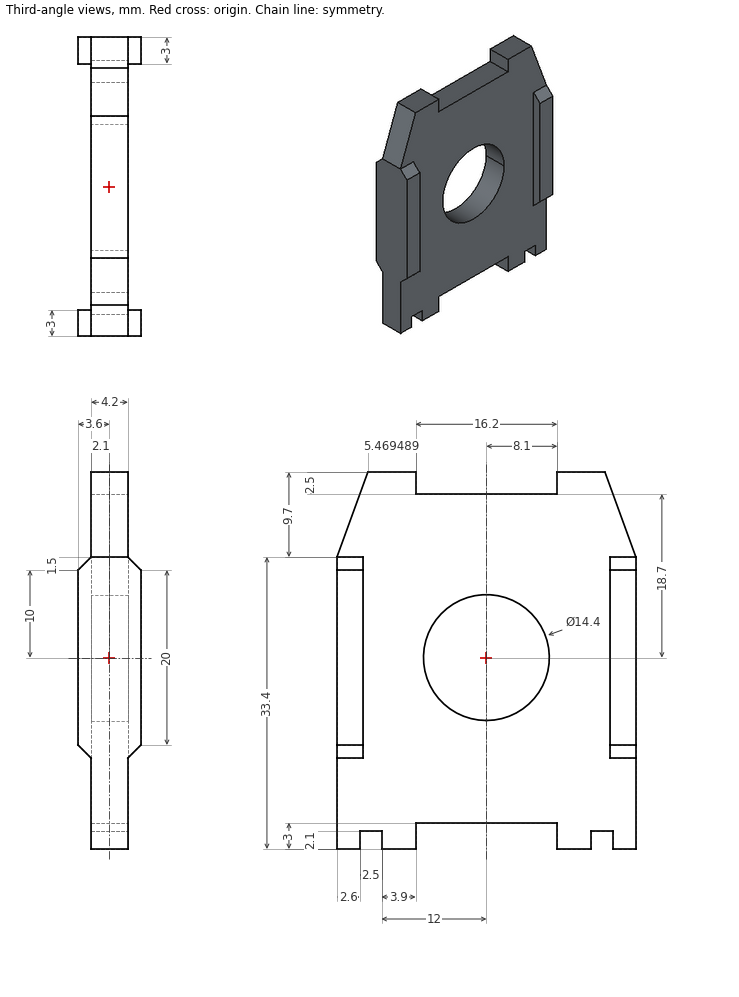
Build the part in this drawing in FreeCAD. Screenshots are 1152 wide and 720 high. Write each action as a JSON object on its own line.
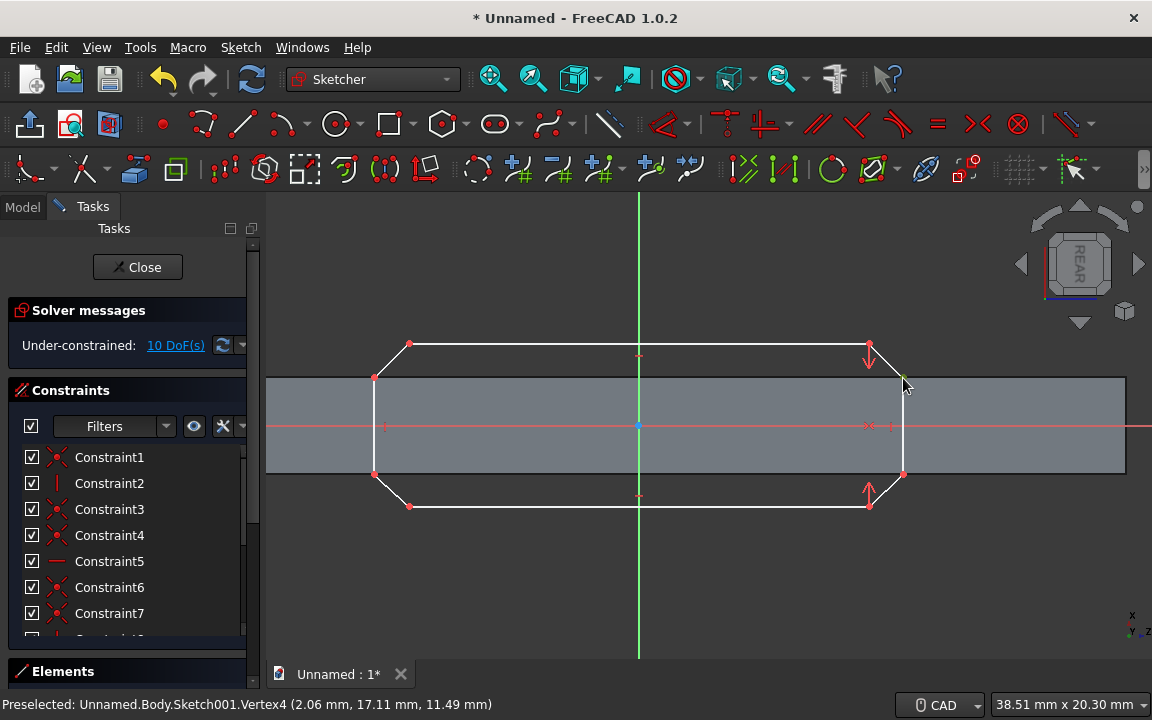
{"action": "left_click", "coordinate": [374, 378]}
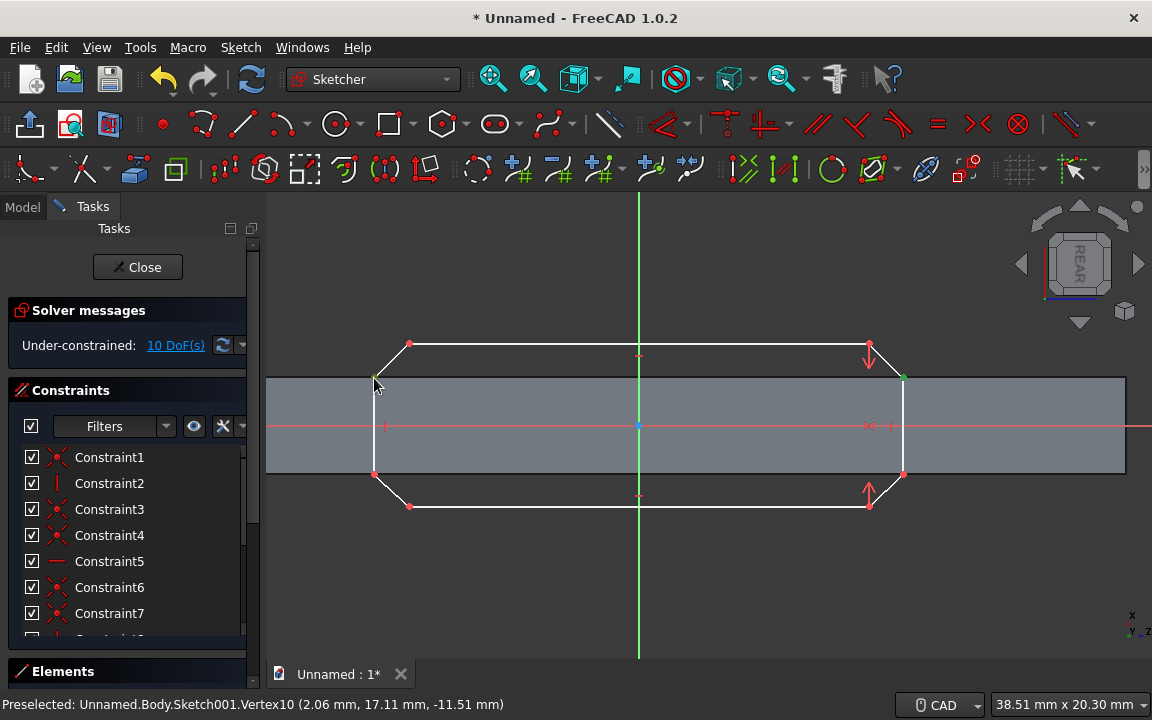
{"action": "left_click", "coordinate": [639, 602]}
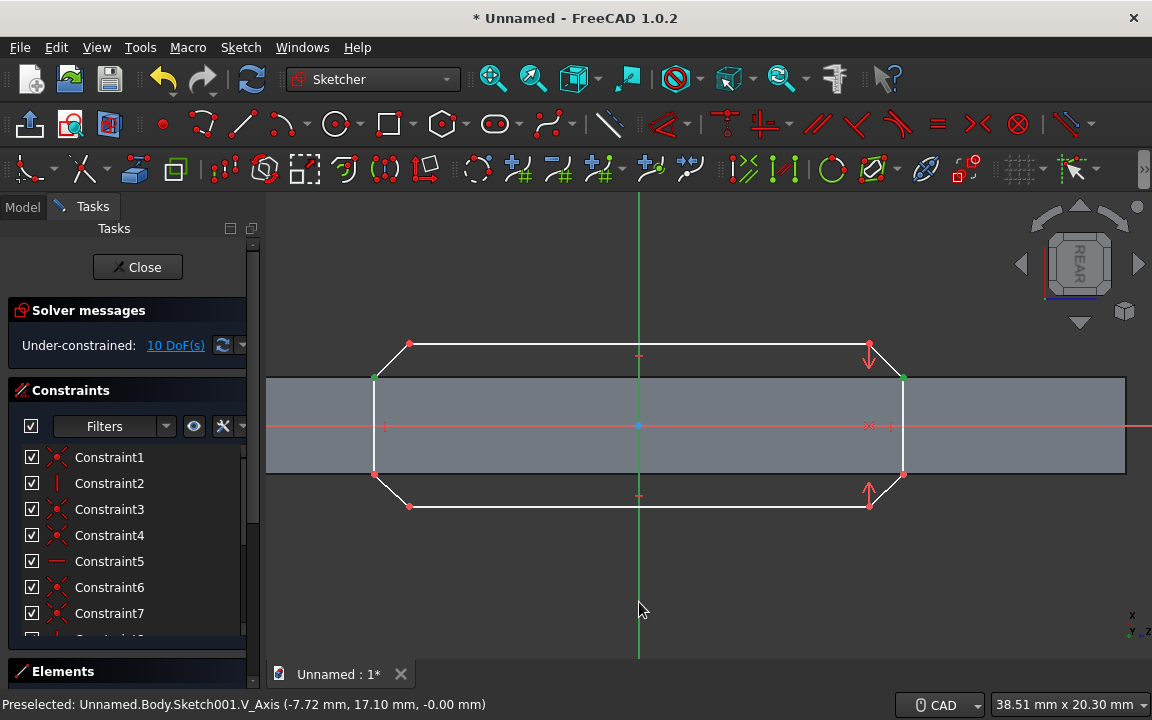
{"action": "key", "text": "s"}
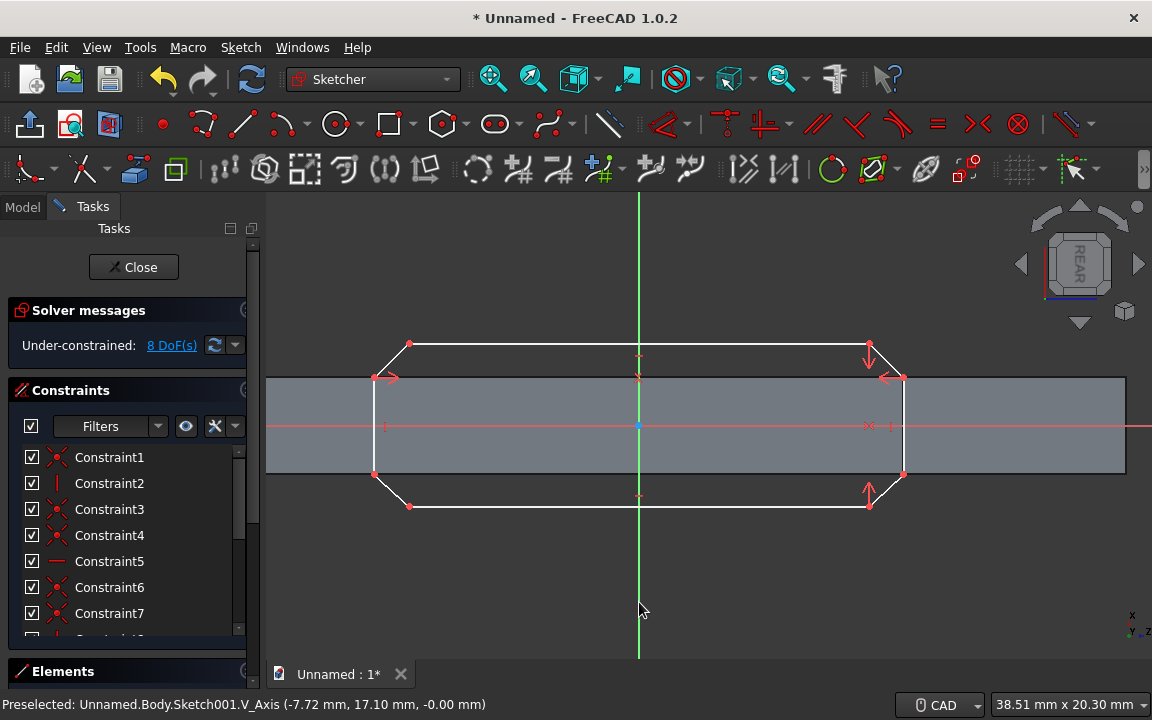
{"action": "left_click", "coordinate": [664, 124]}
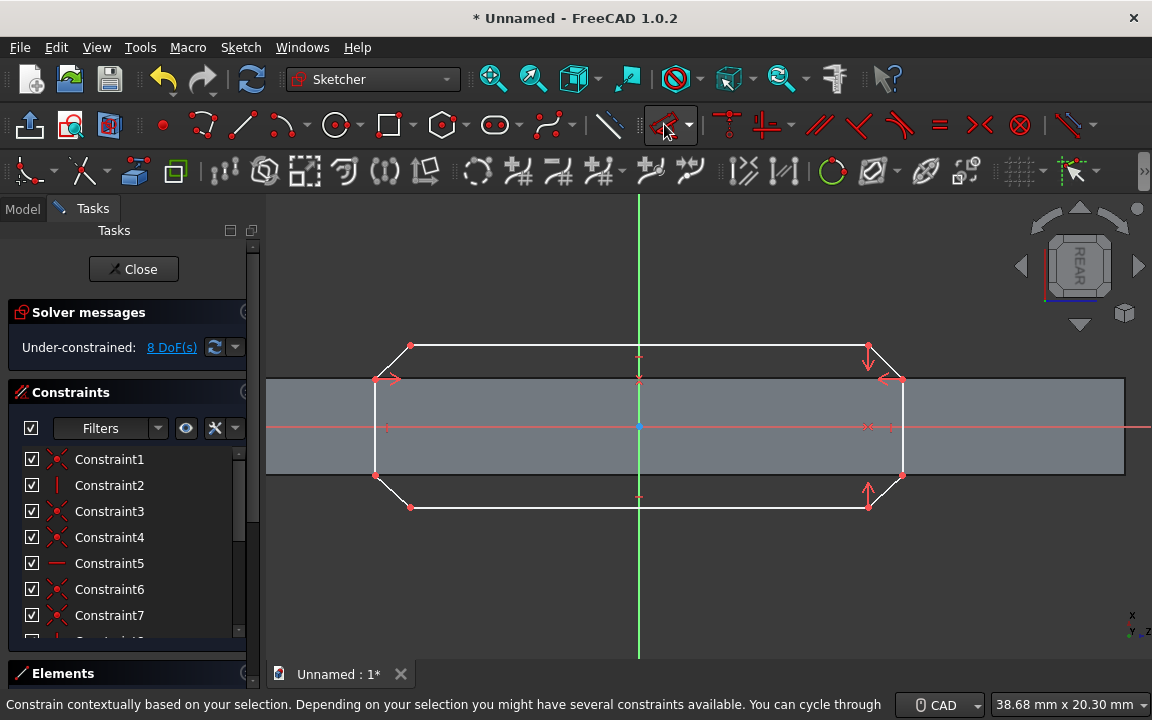
{"action": "left_click", "coordinate": [731, 345]}
{"action": "left_click", "coordinate": [534, 311]}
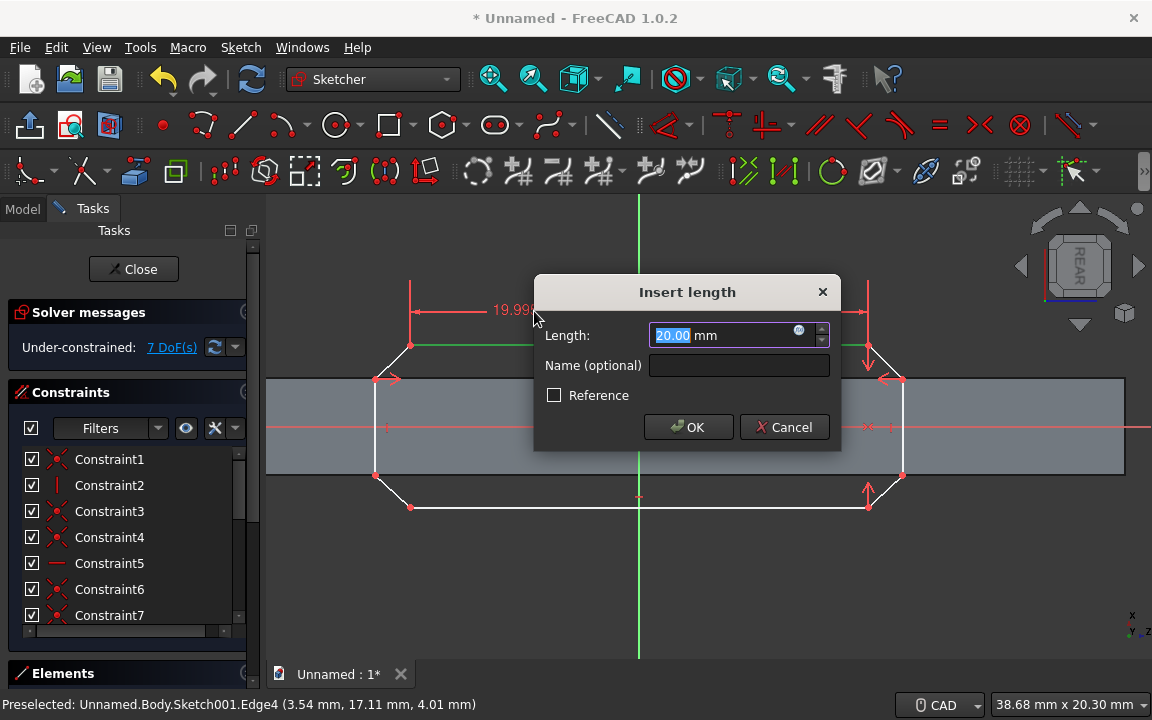
{"action": "type", "text": "20"}
{"action": "key", "text": "Return"}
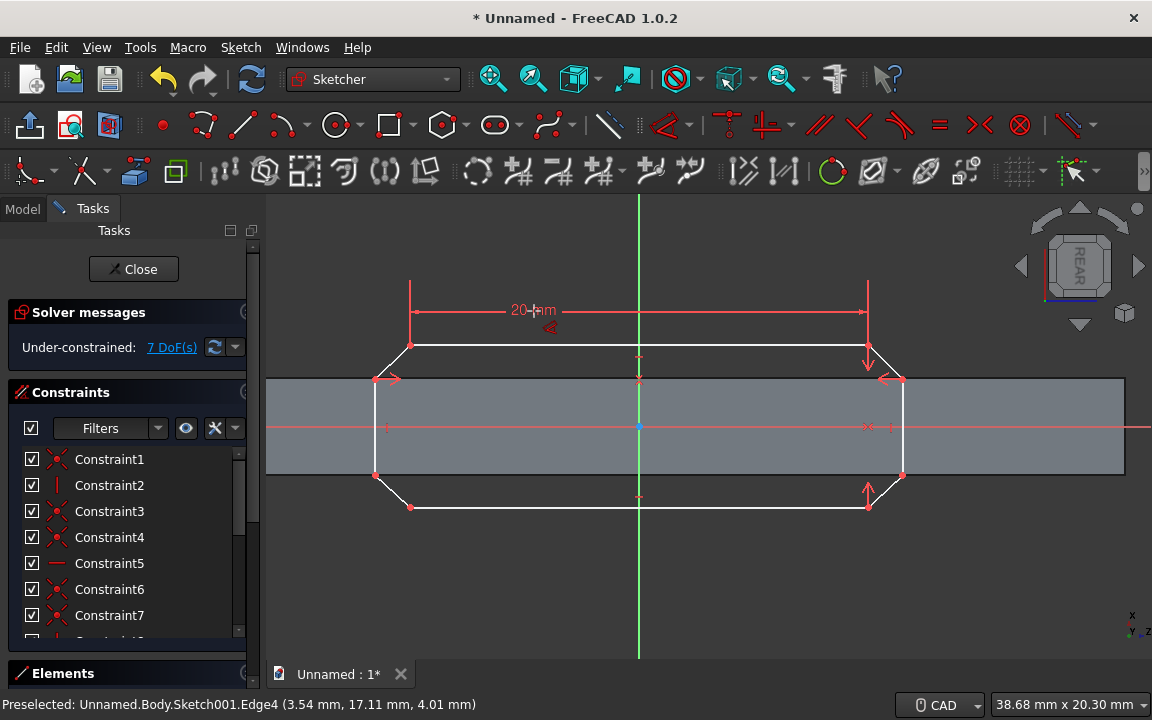
{"action": "left_click", "coordinate": [548, 508]}
{"action": "left_click", "coordinate": [534, 542]}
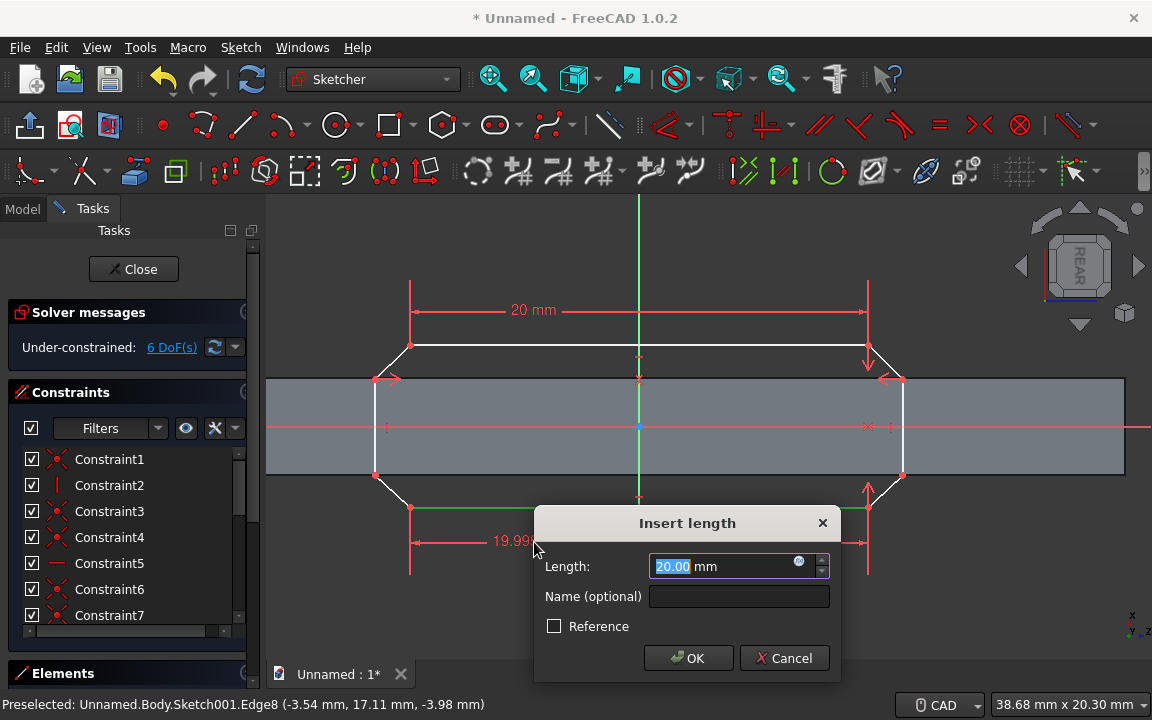
{"action": "type", "text": "20"}
{"action": "key", "text": "Return"}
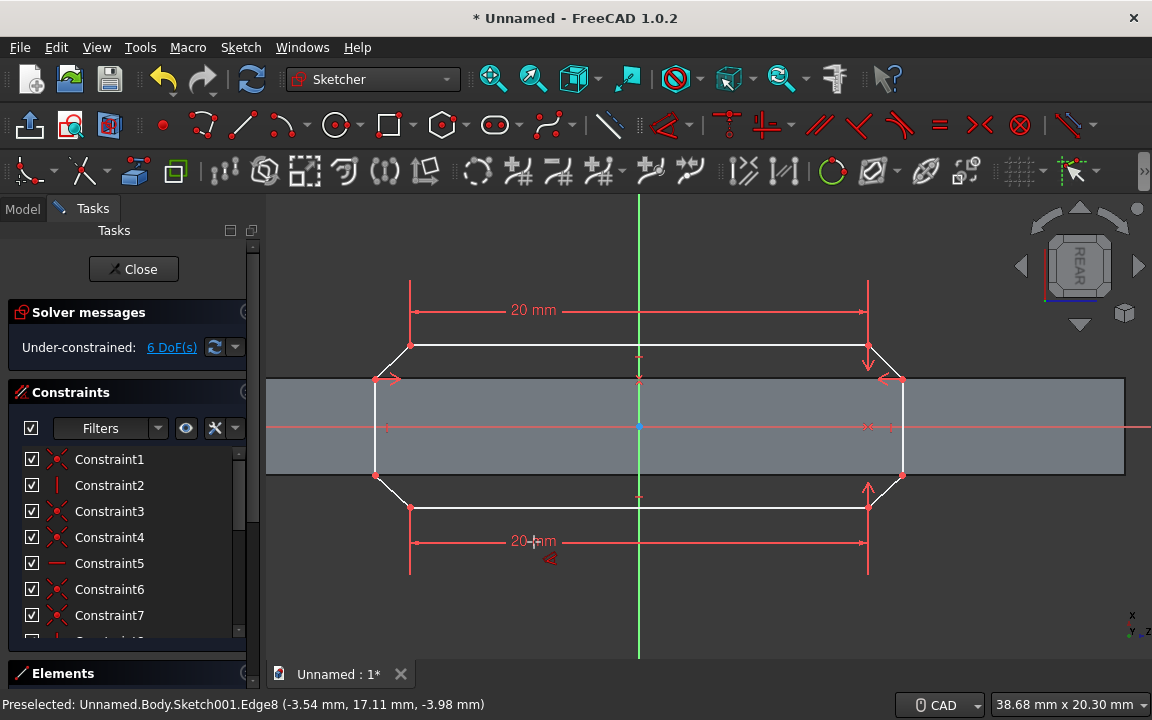
{"action": "left_click", "coordinate": [903, 447]}
{"action": "left_click", "coordinate": [937, 405]}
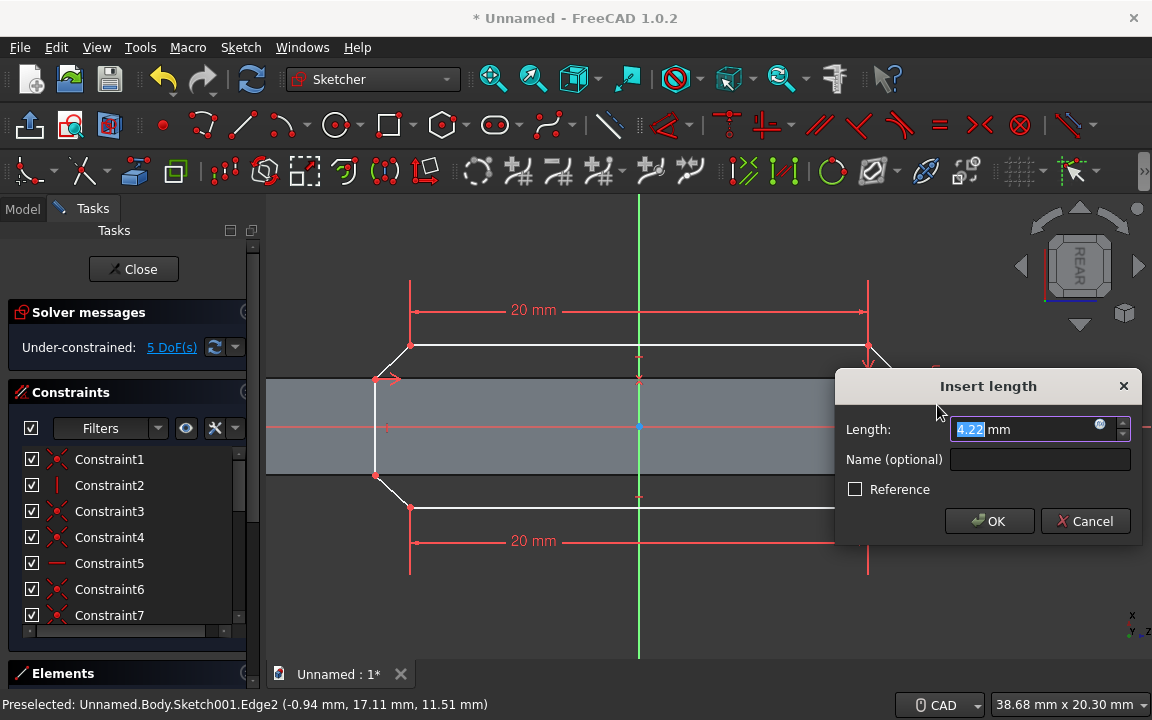
{"action": "type", "text": "4.2"}
{"action": "key", "text": "Return"}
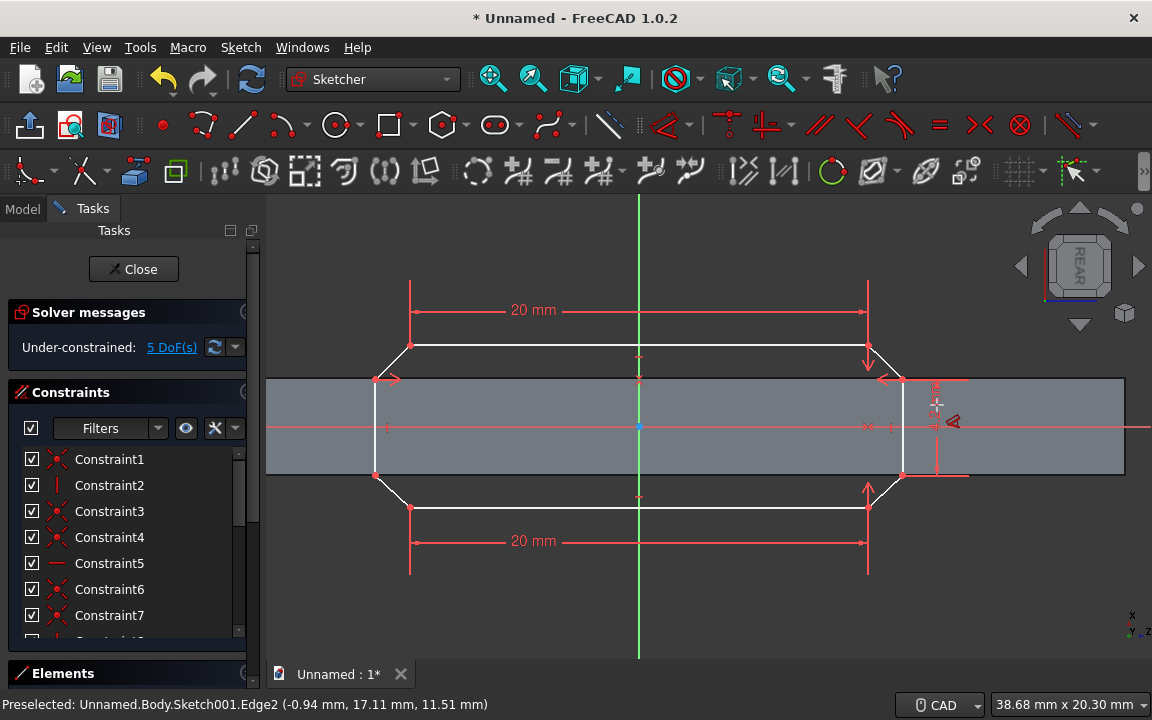
{"action": "left_click", "coordinate": [375, 408]}
{"action": "left_click", "coordinate": [341, 406]}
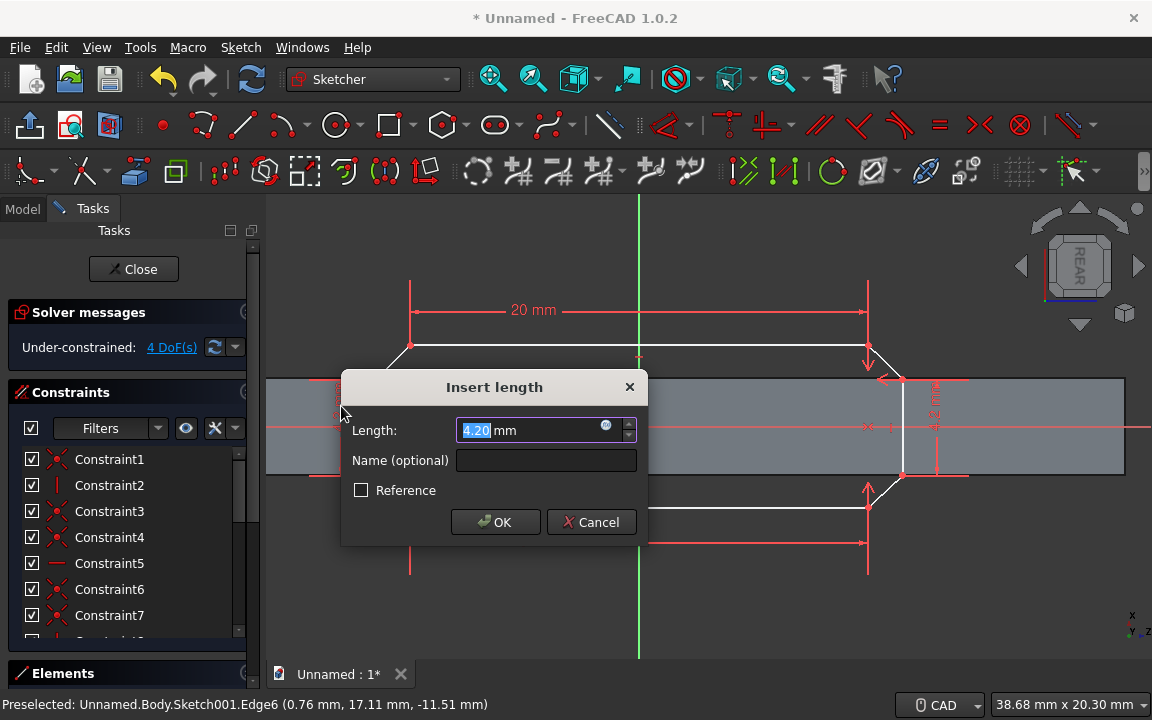
{"action": "type", "text": "4.2"}
{"action": "key", "text": "Return"}